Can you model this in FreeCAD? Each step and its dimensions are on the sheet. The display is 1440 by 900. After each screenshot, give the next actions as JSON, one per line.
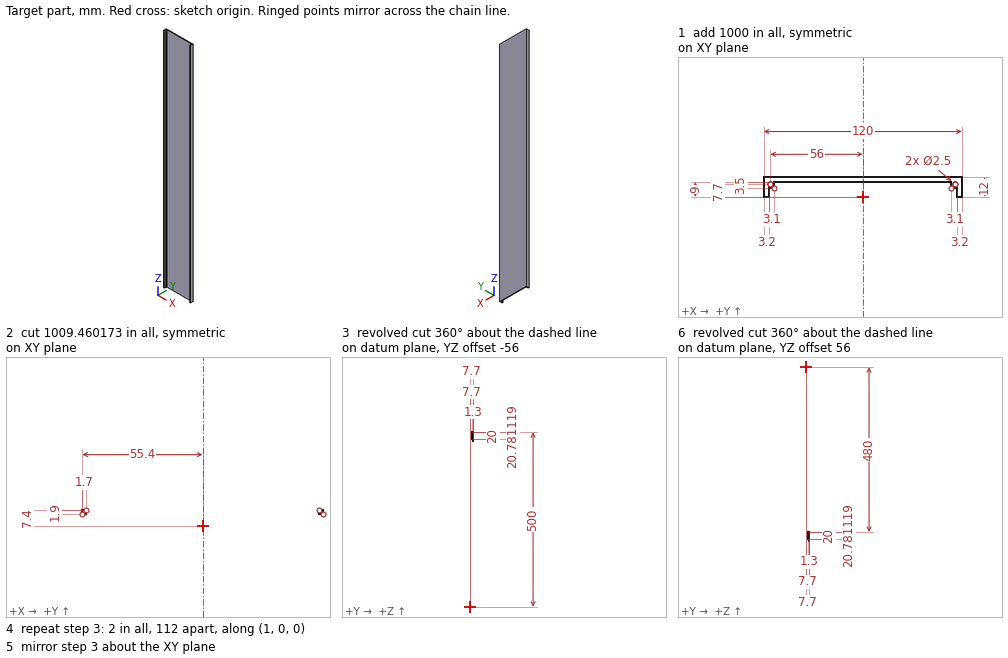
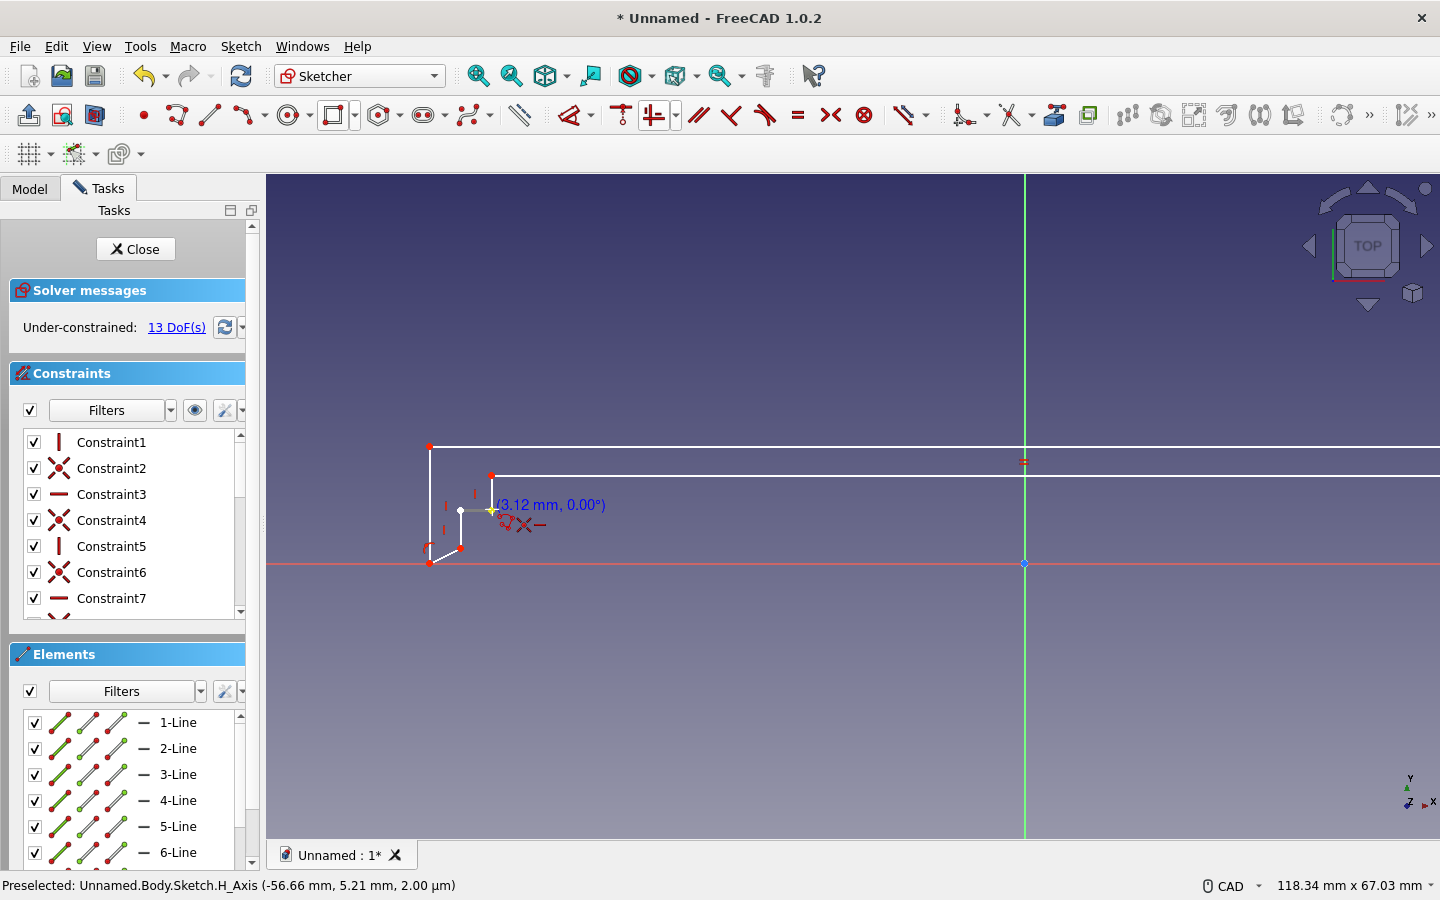
{"action": "left_click", "coordinate": [492, 510]}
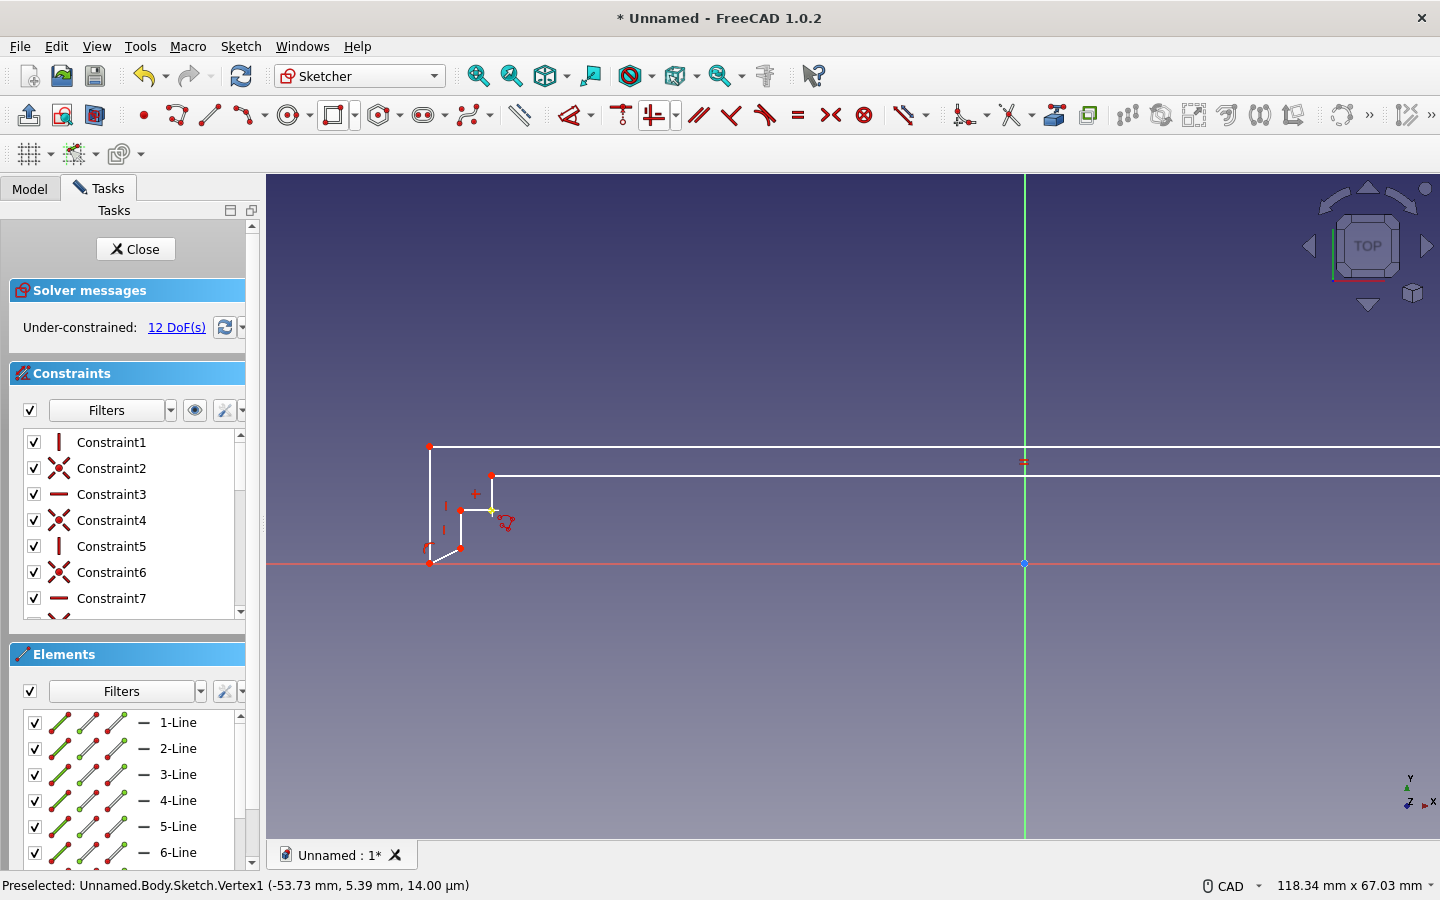
{"action": "key", "text": "g c"}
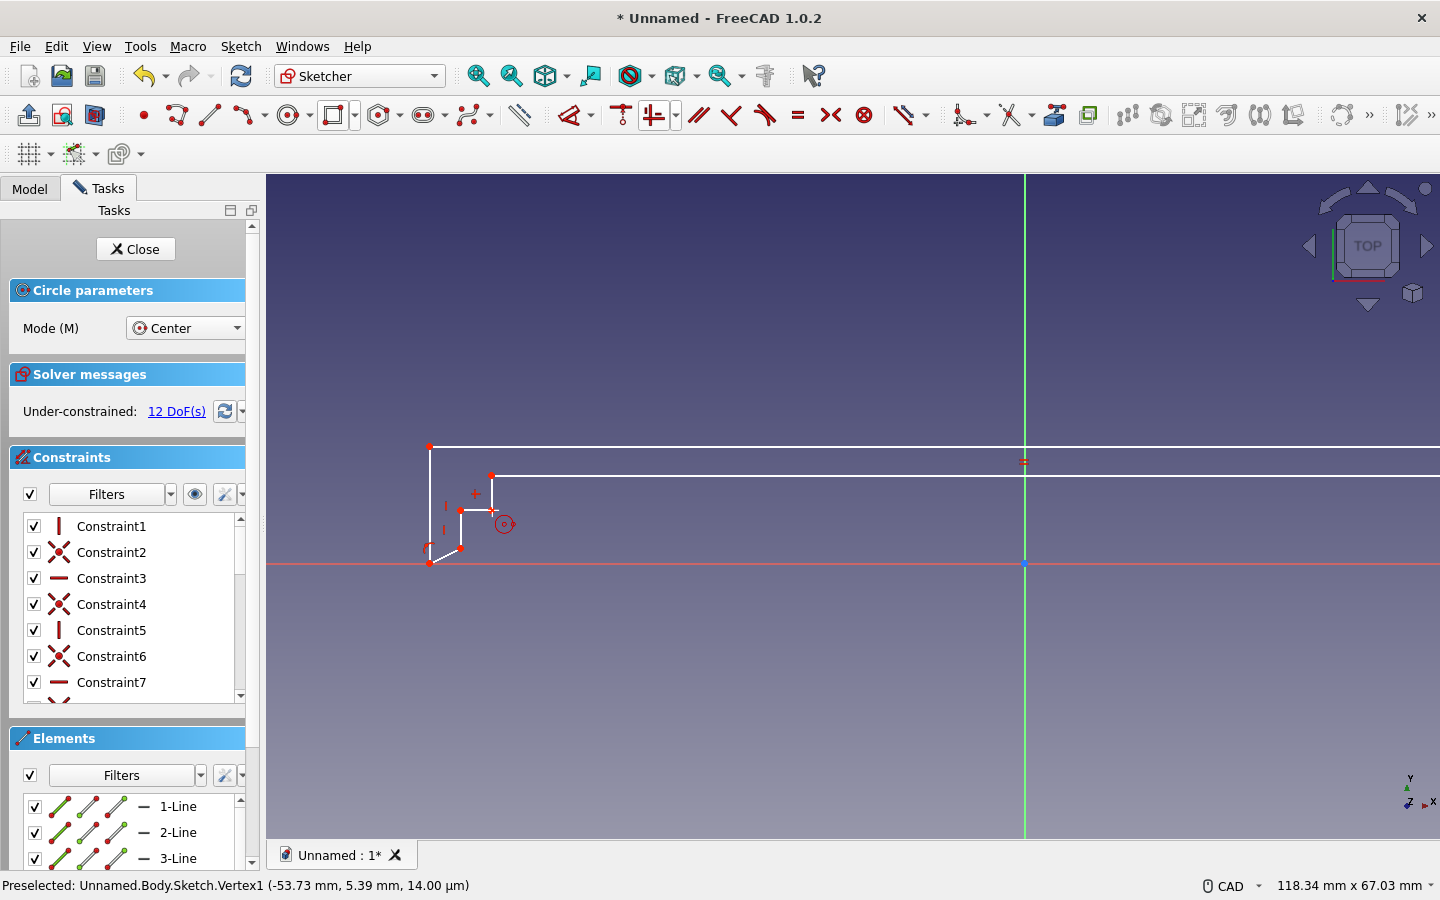
{"action": "scroll", "coordinate": [469, 488], "scroll_direction": "up", "scroll_amount": 4}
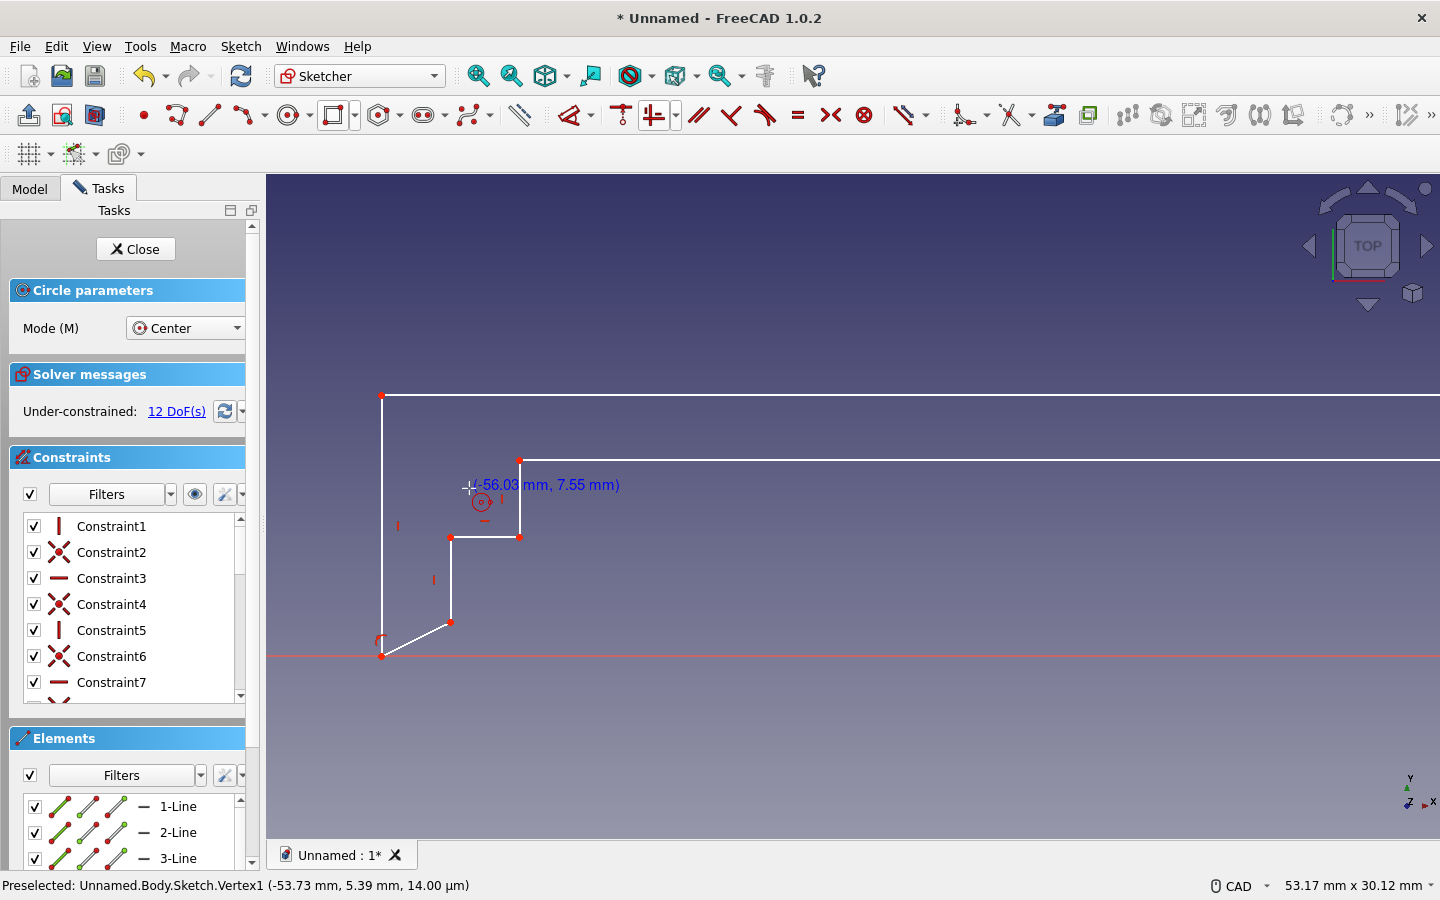
{"action": "scroll", "coordinate": [483, 501], "scroll_direction": "down", "scroll_amount": 7}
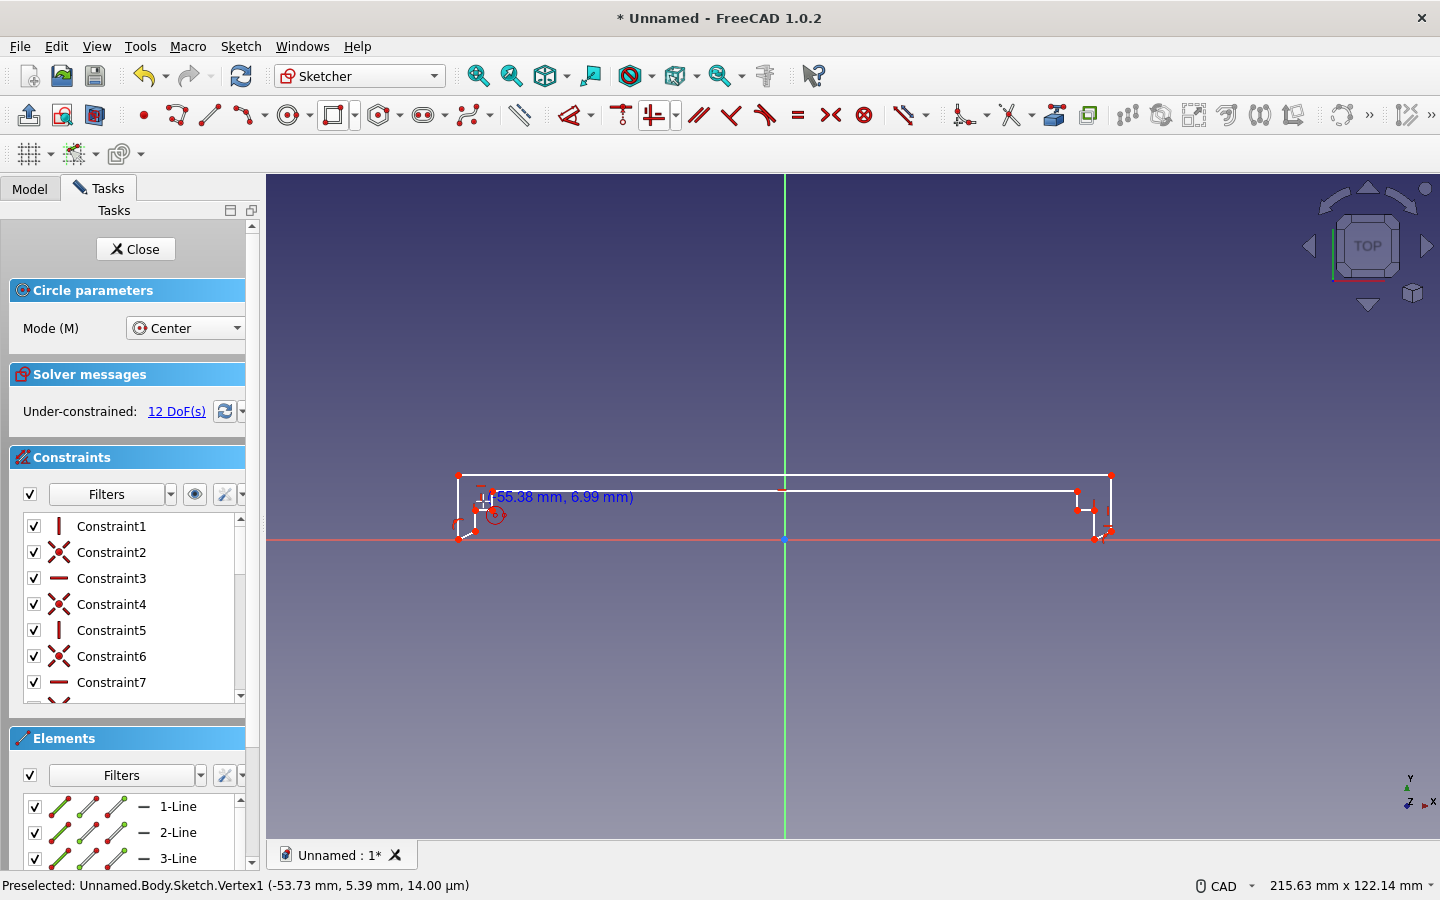
{"action": "scroll", "coordinate": [480, 498], "scroll_direction": "up", "scroll_amount": 2}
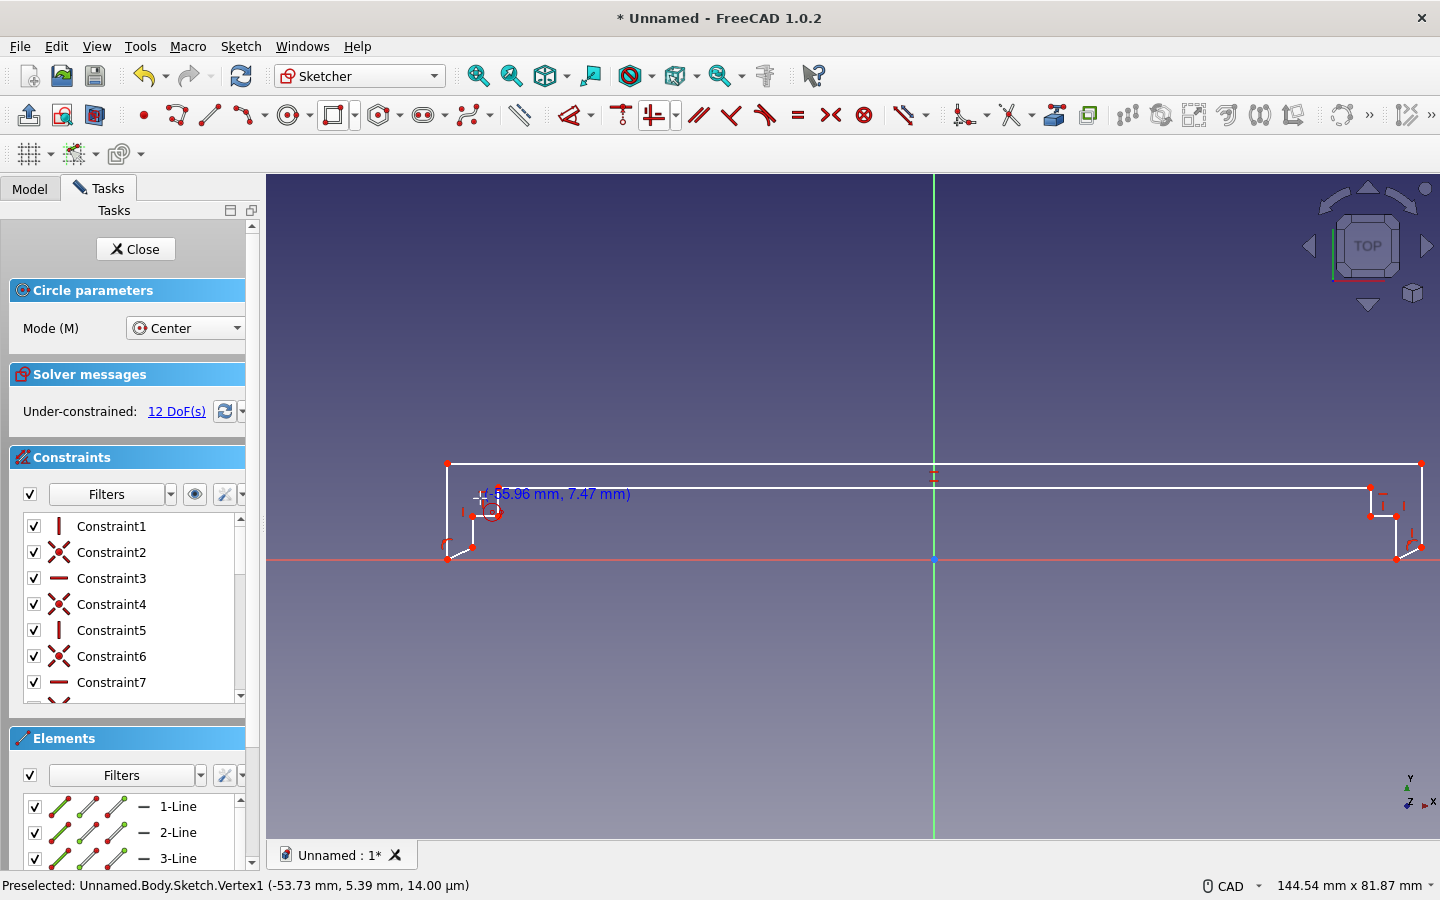
{"action": "left_click", "coordinate": [480, 497]}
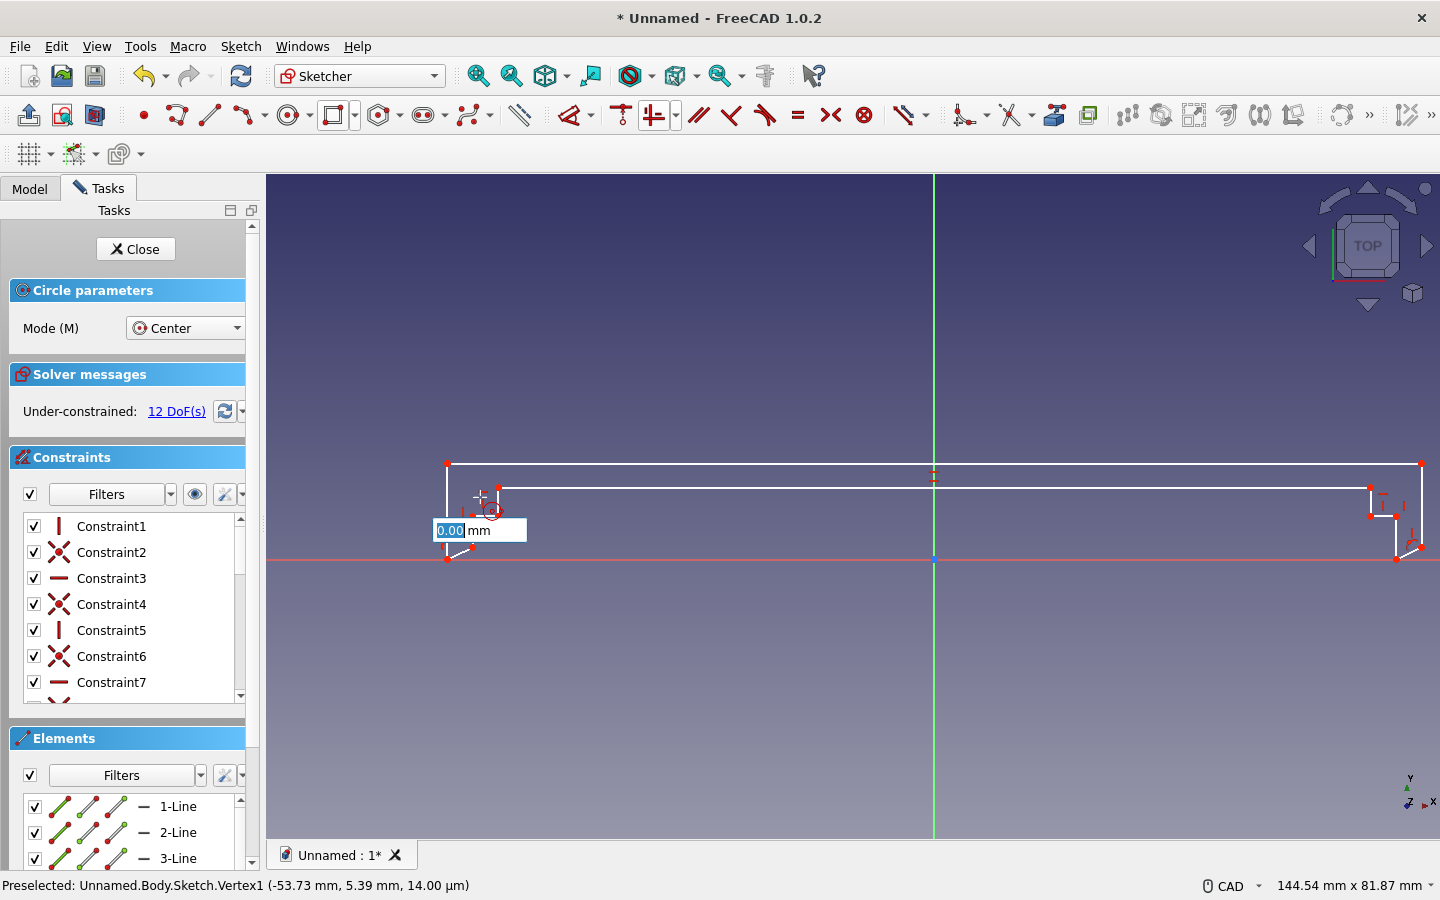
{"action": "scroll", "coordinate": [472, 490], "scroll_direction": "up", "scroll_amount": 3}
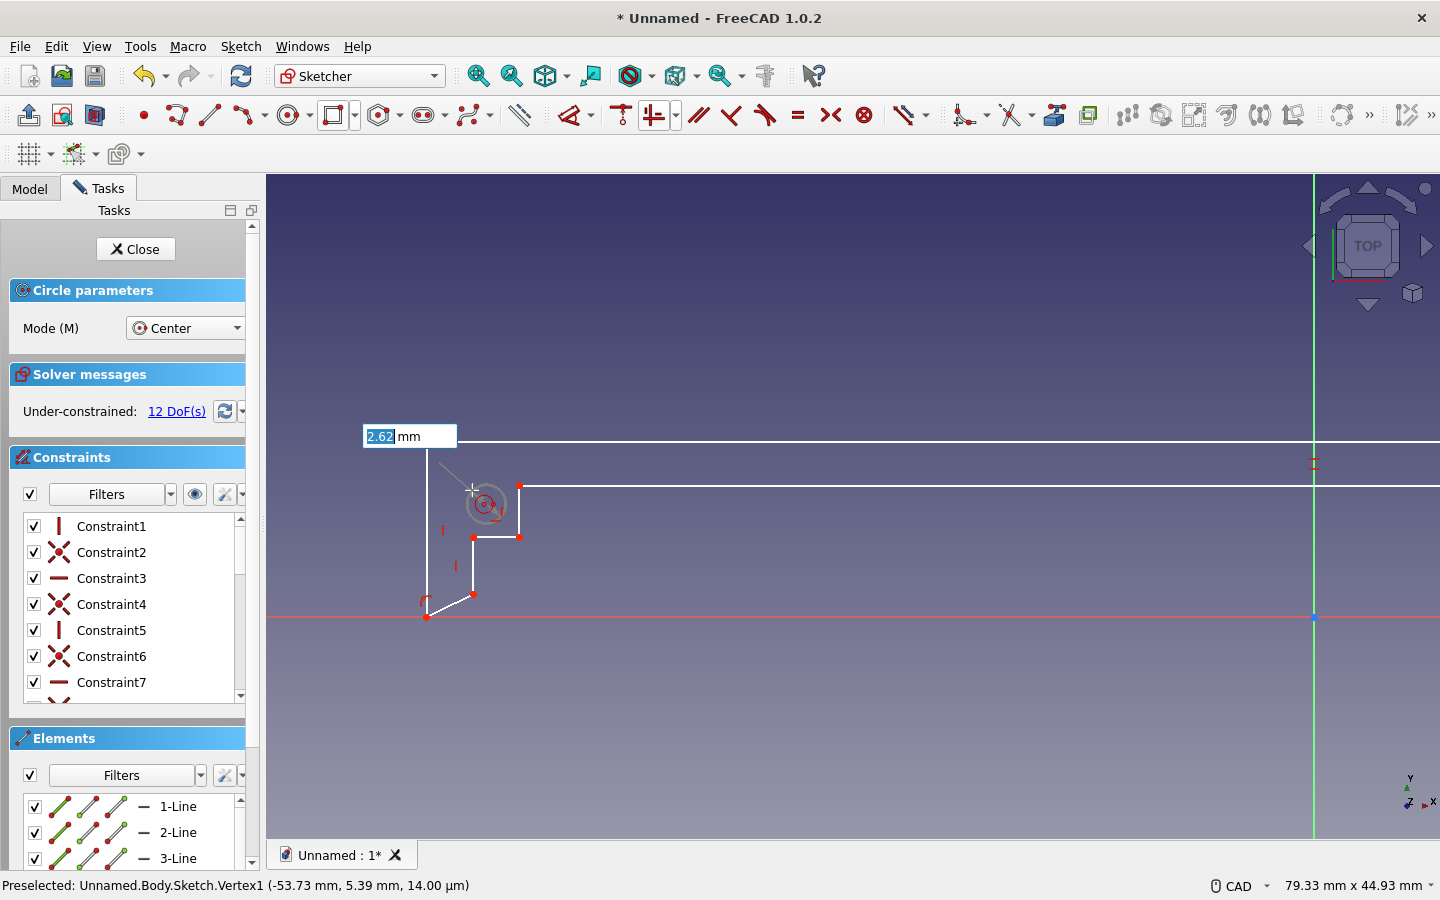
{"action": "left_click", "coordinate": [473, 490]}